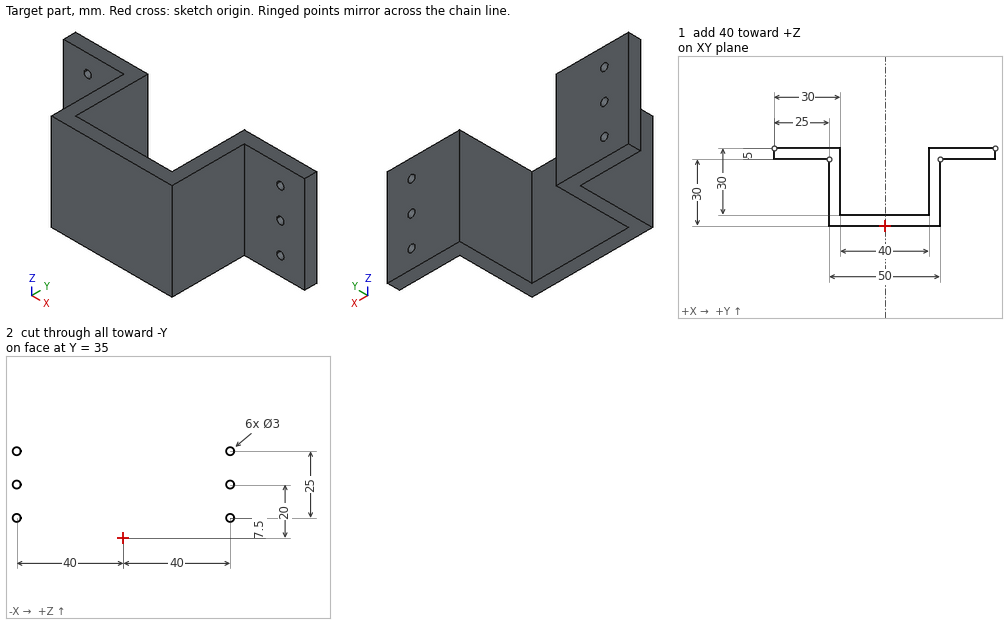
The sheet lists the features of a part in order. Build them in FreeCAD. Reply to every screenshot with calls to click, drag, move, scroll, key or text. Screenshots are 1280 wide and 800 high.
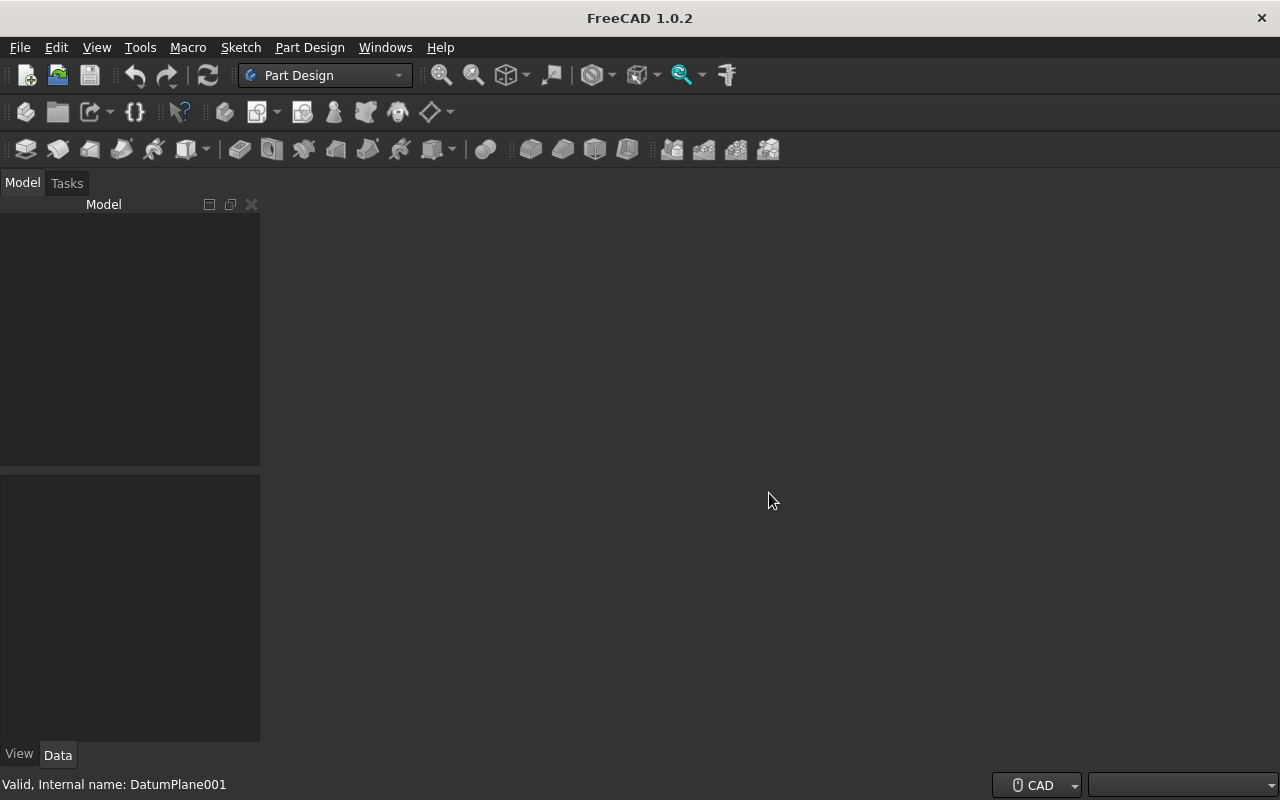
click(26, 76)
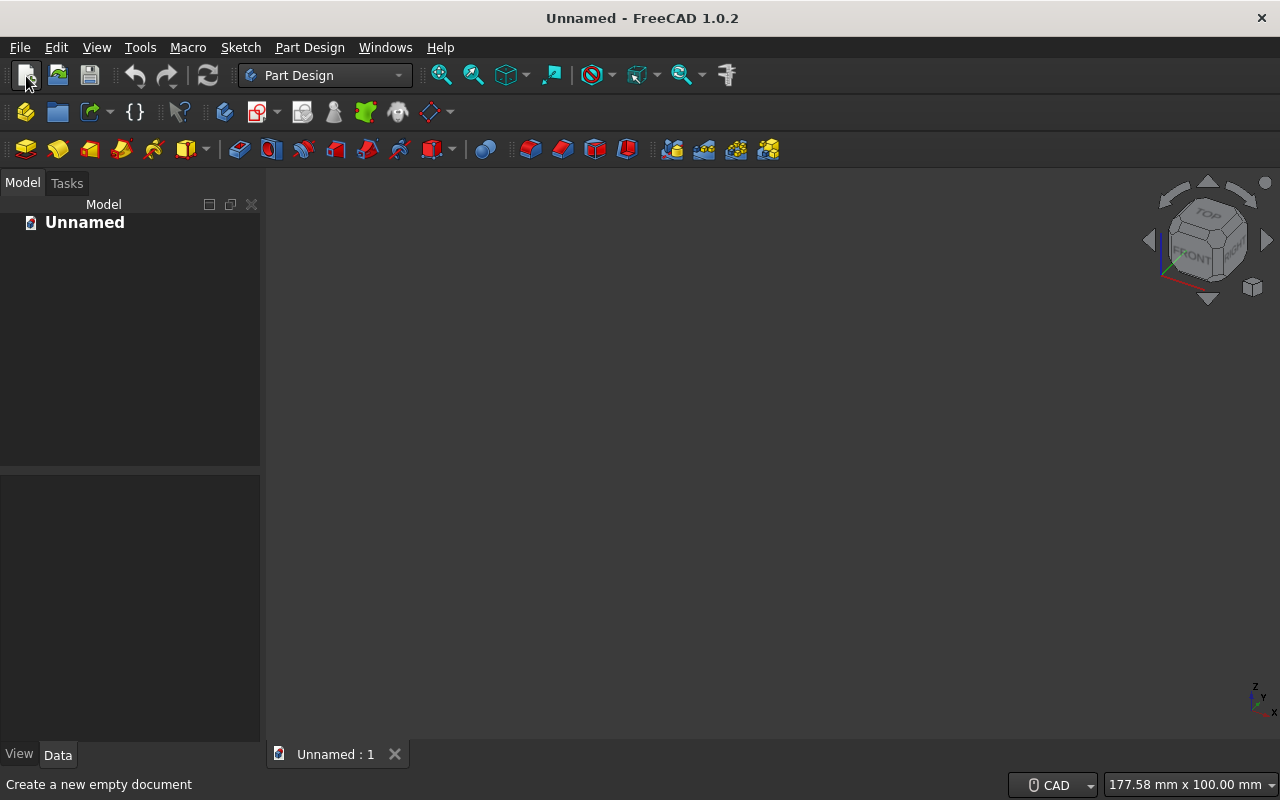
click(258, 112)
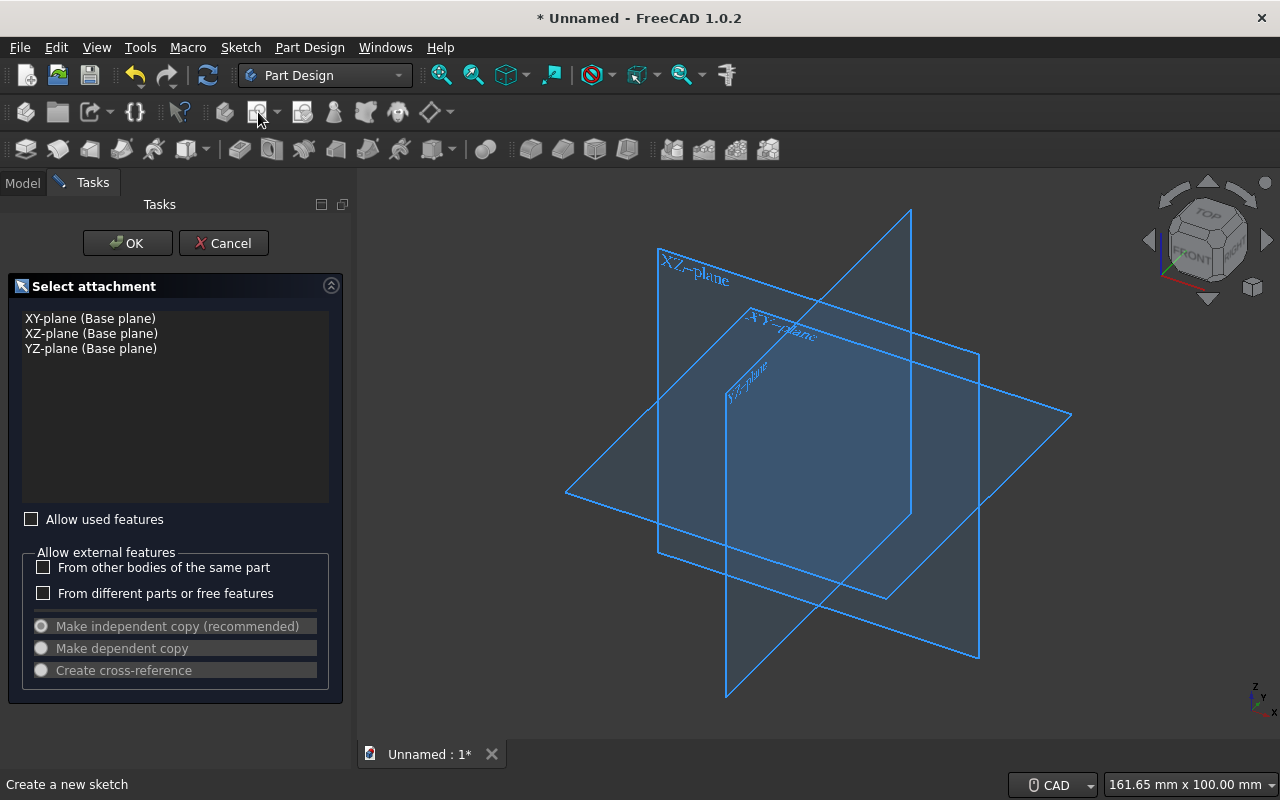
click(82, 318)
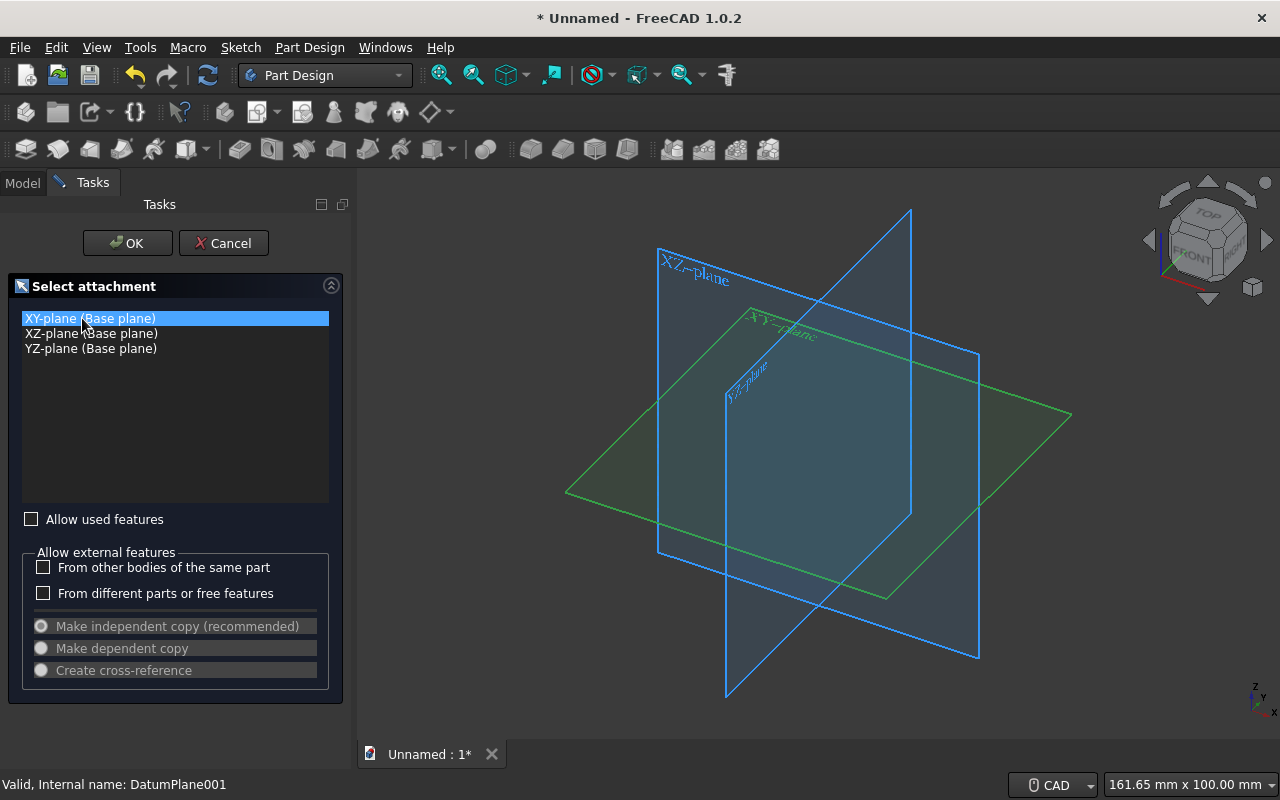
click(128, 243)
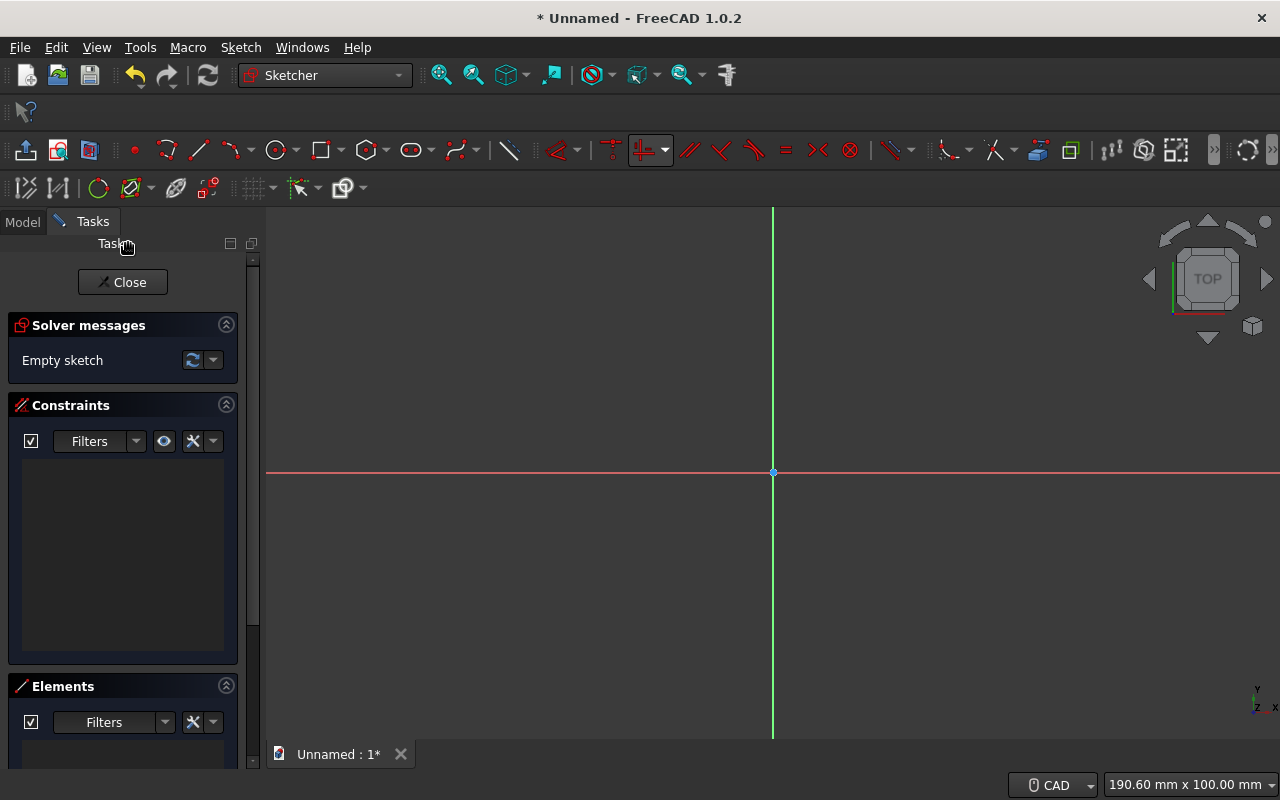
key(g)
key(m)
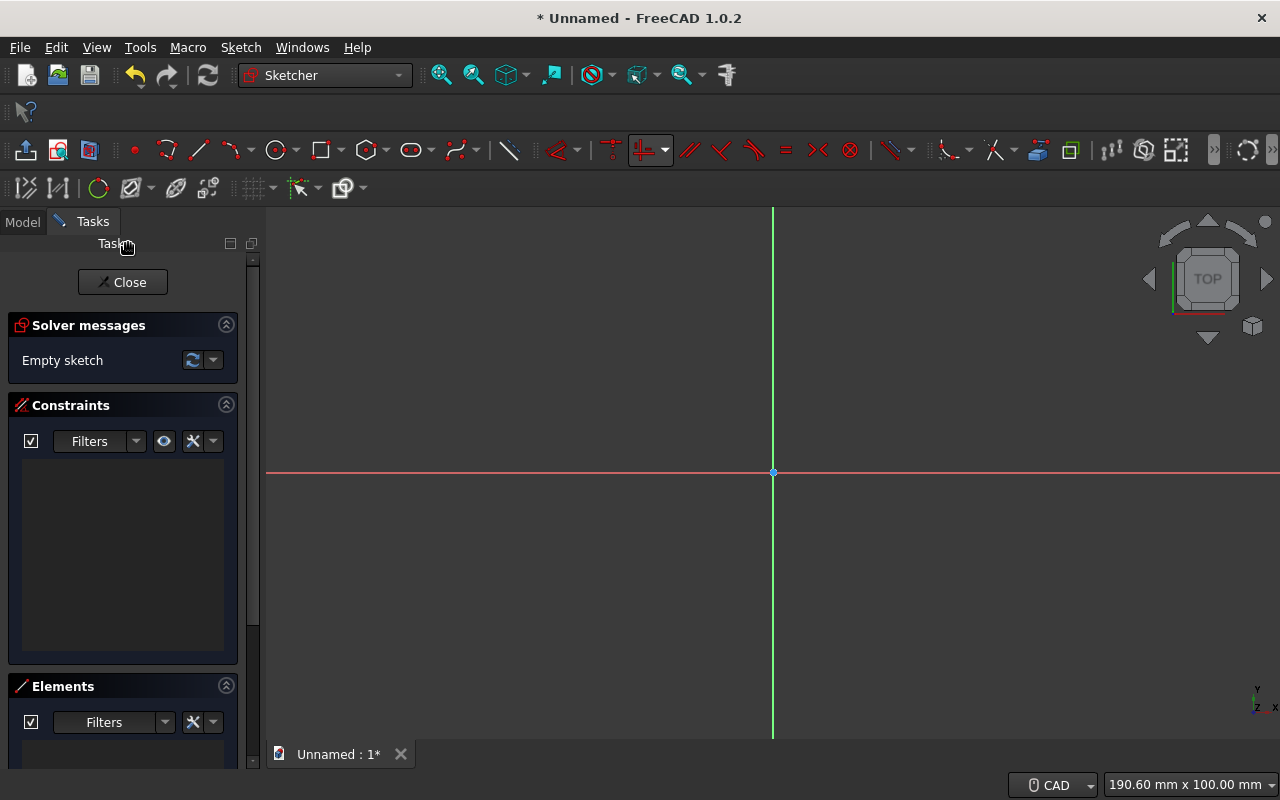
click(879, 446)
click(667, 446)
click(667, 287)
click(507, 287)
click(507, 313)
click(640, 313)
click(640, 473)
click(906, 464)
click(906, 313)
click(1039, 313)
click(1039, 287)
click(879, 287)
click(879, 447)
key(Escape)
key(Escape)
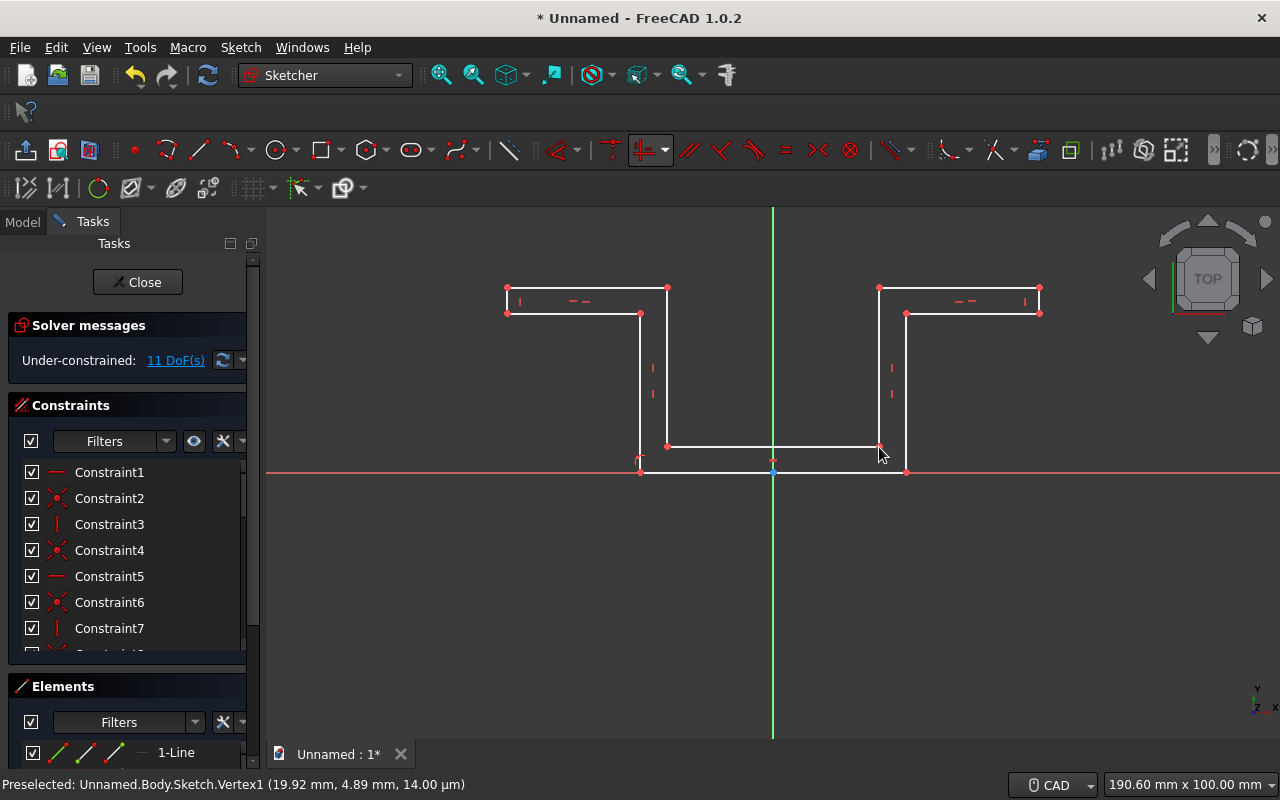
click(640, 314)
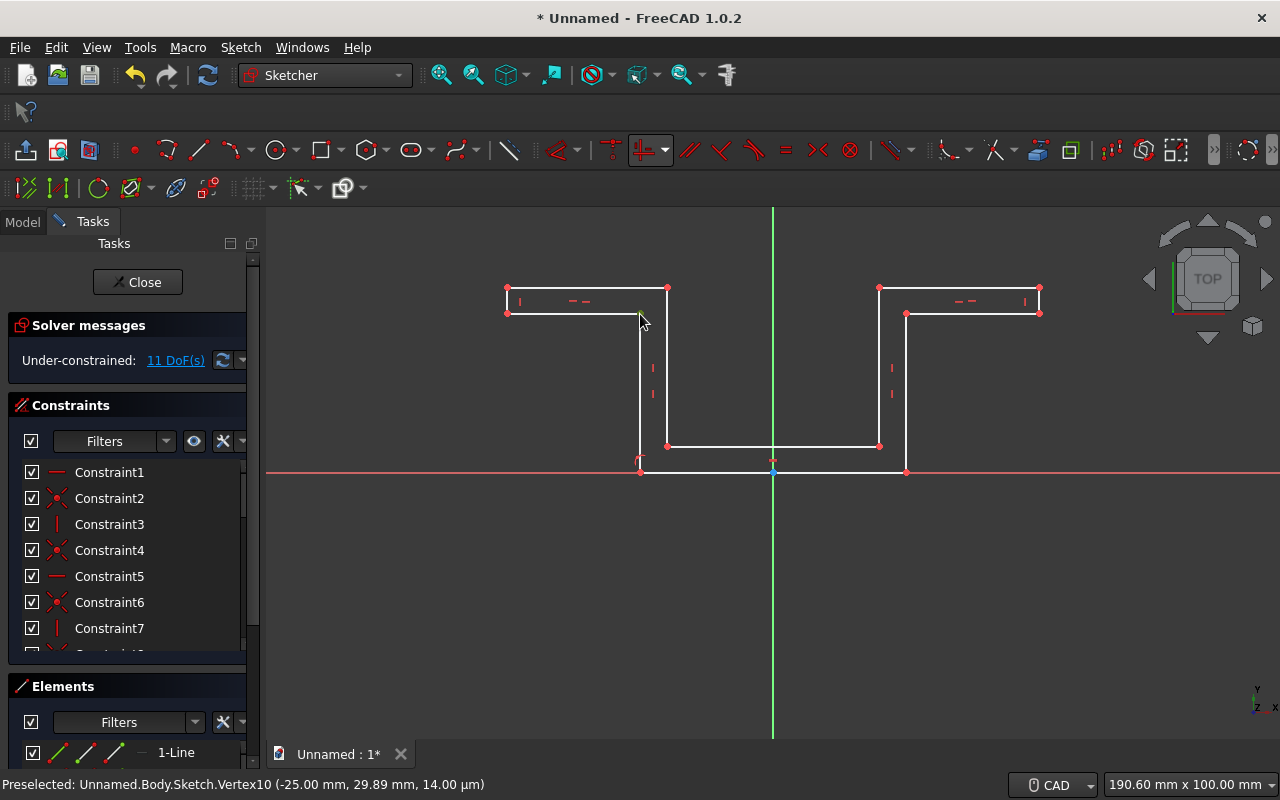
click(906, 314)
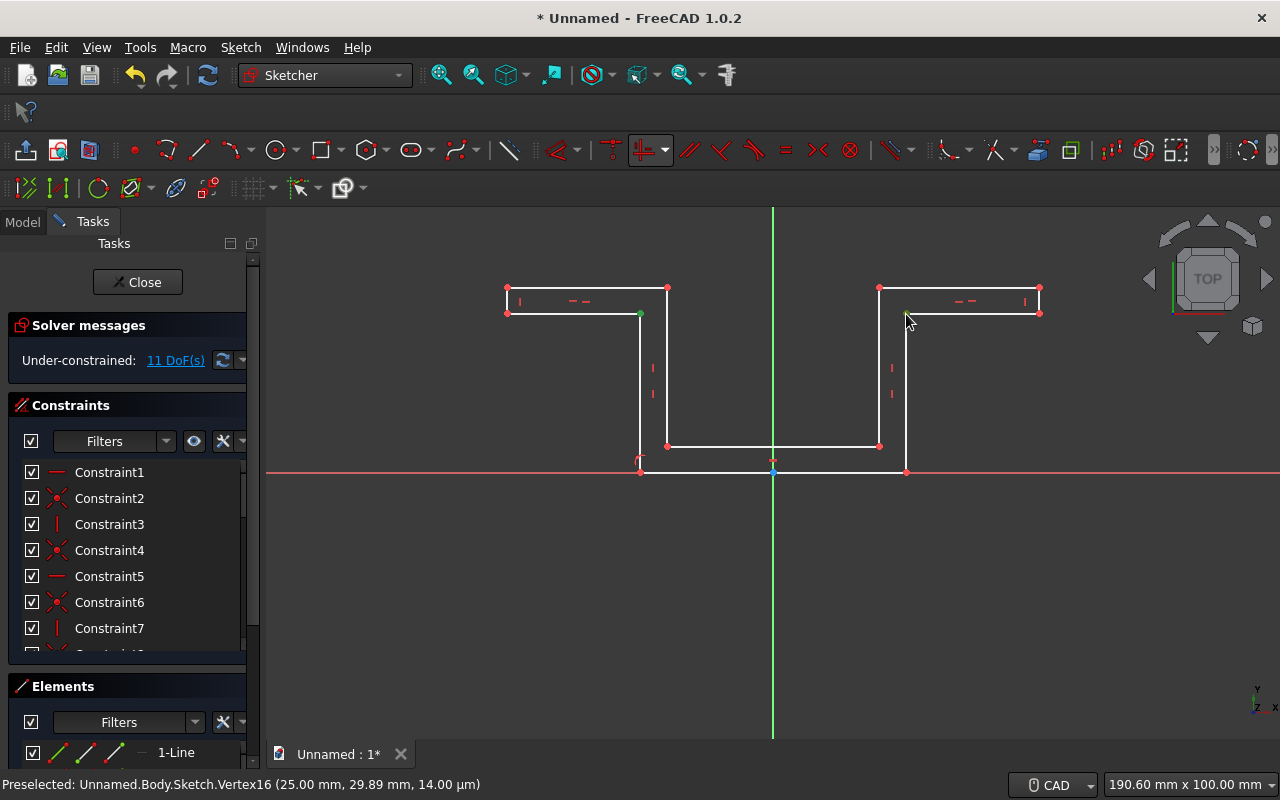
click(773, 677)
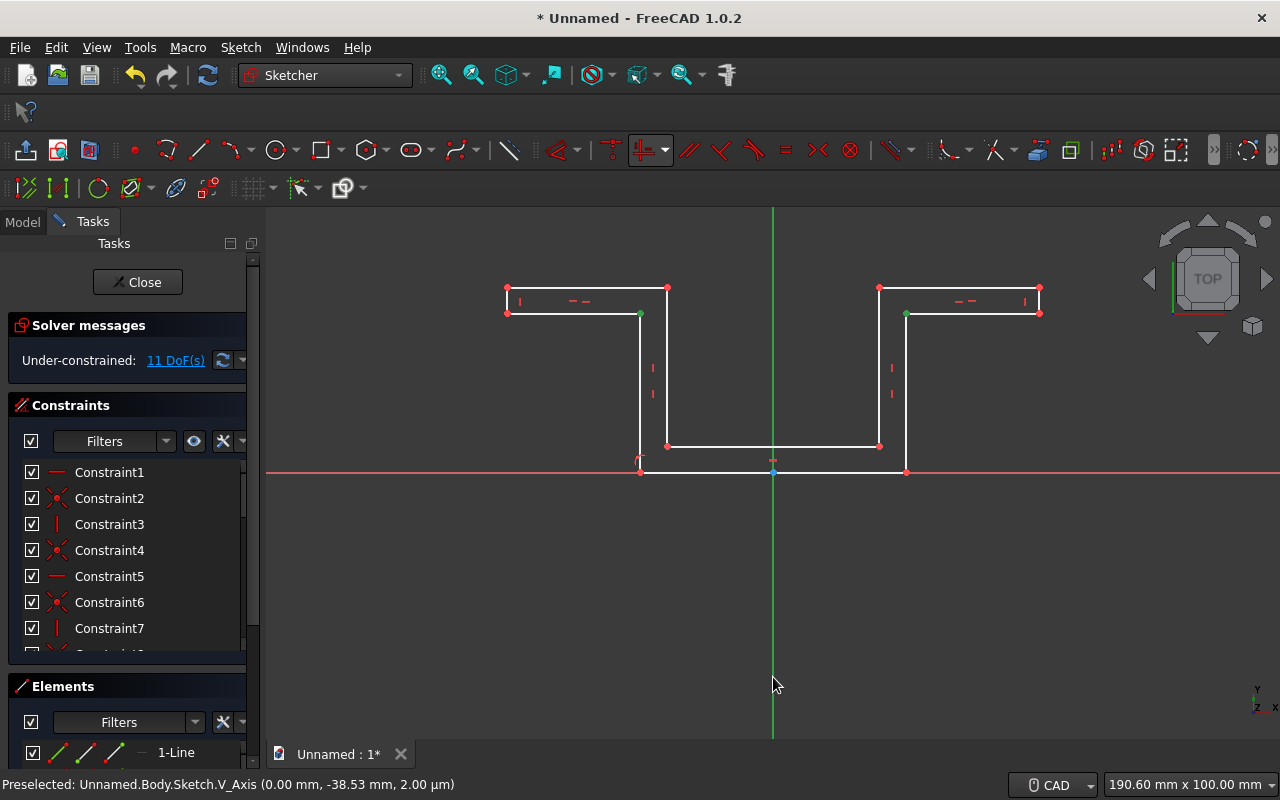
key(s)